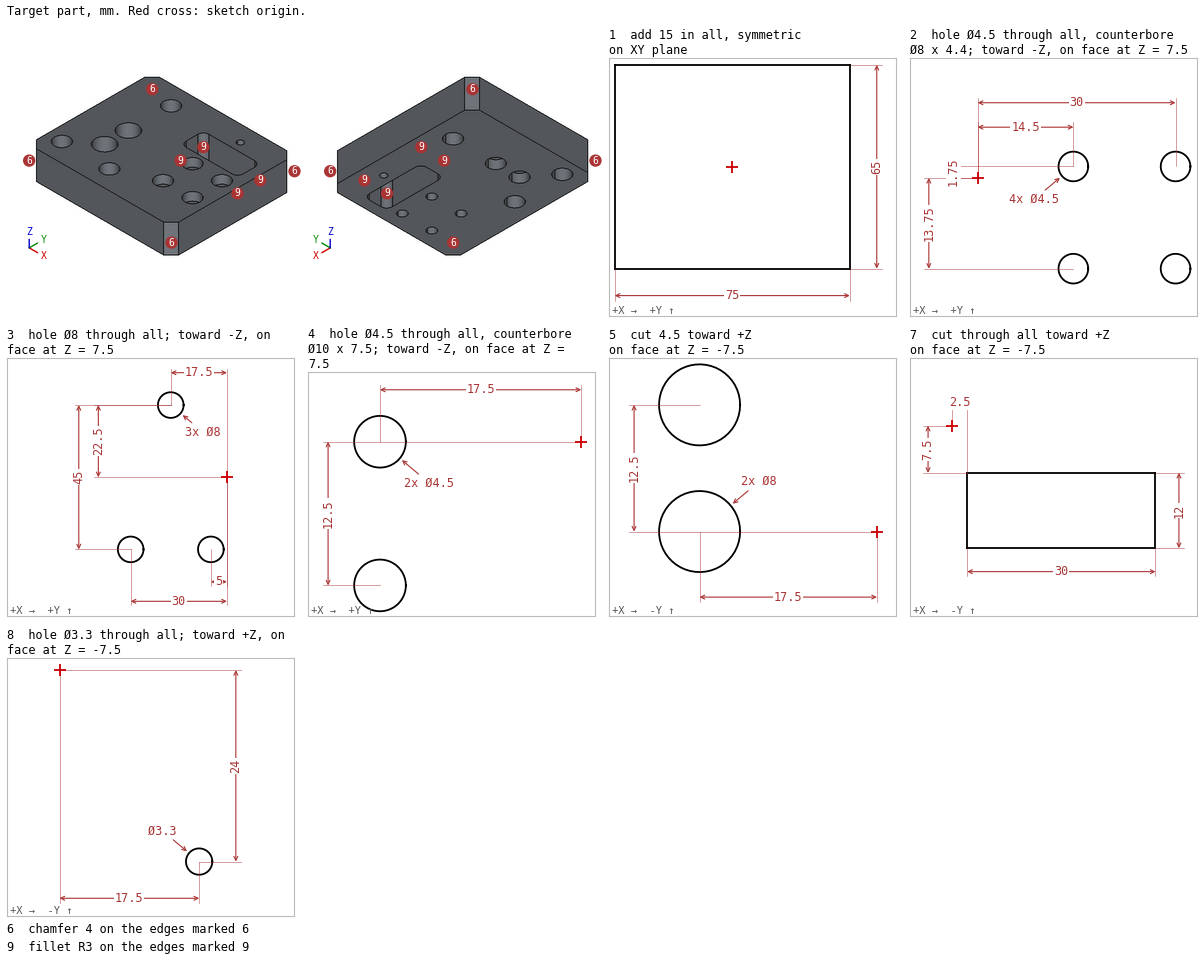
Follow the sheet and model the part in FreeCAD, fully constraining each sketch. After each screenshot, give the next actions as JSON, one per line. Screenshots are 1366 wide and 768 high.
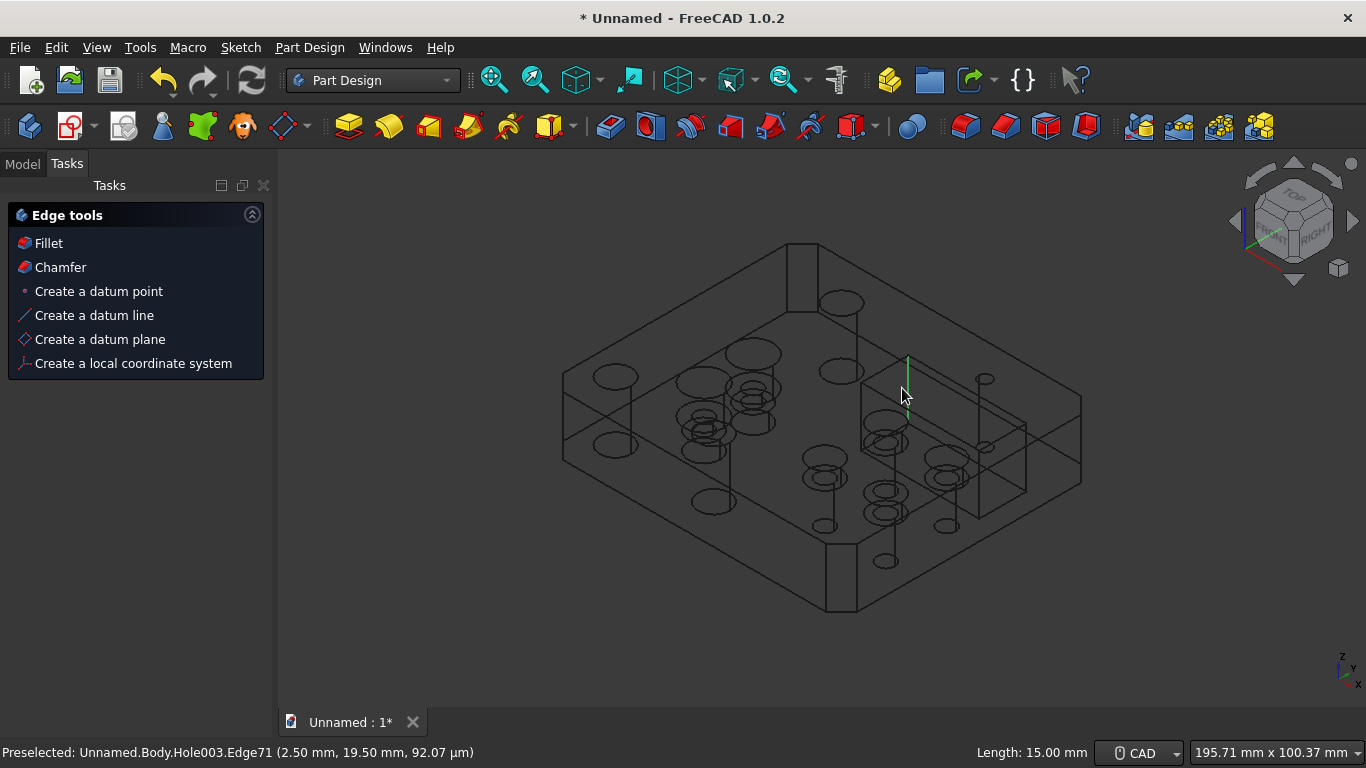
{"action": "left_click", "coordinate": [861, 409], "text": "ctrl"}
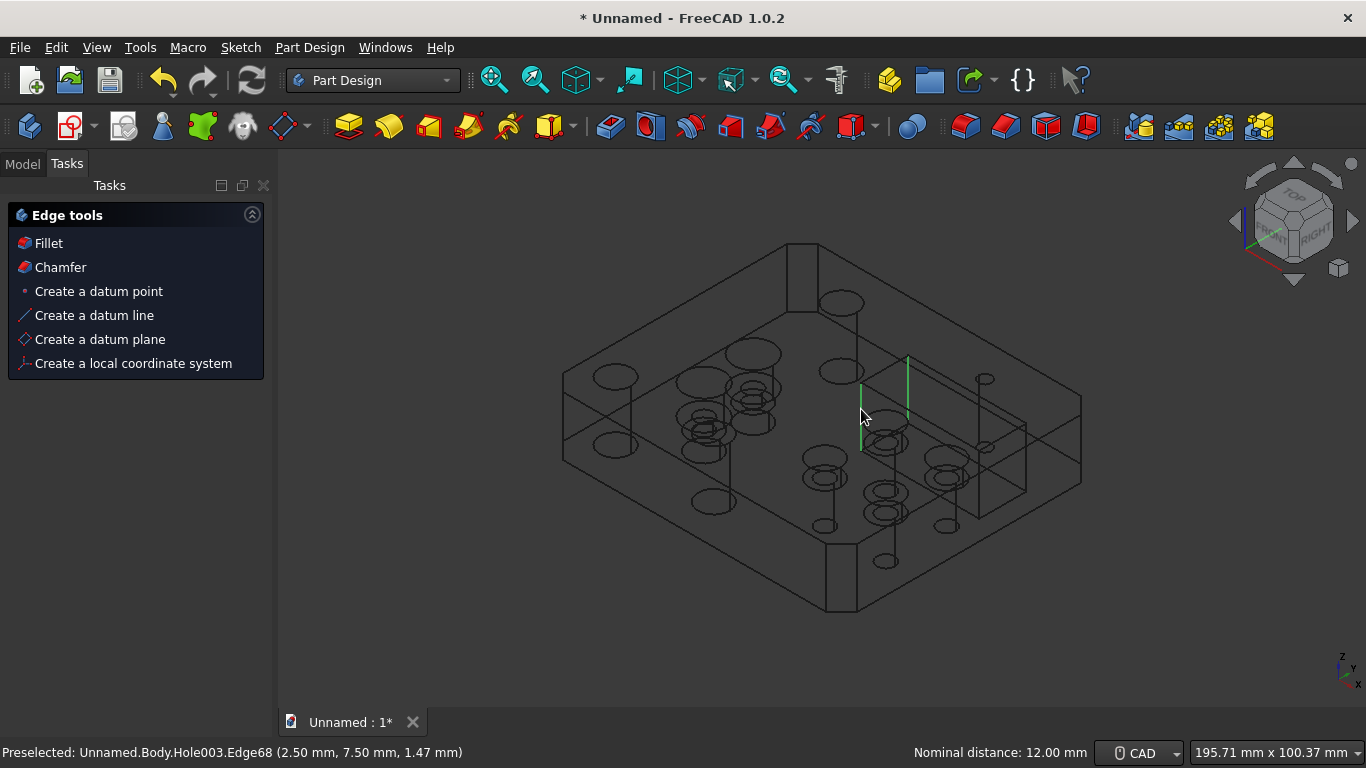
{"action": "left_click", "coordinate": [979, 484], "text": "ctrl"}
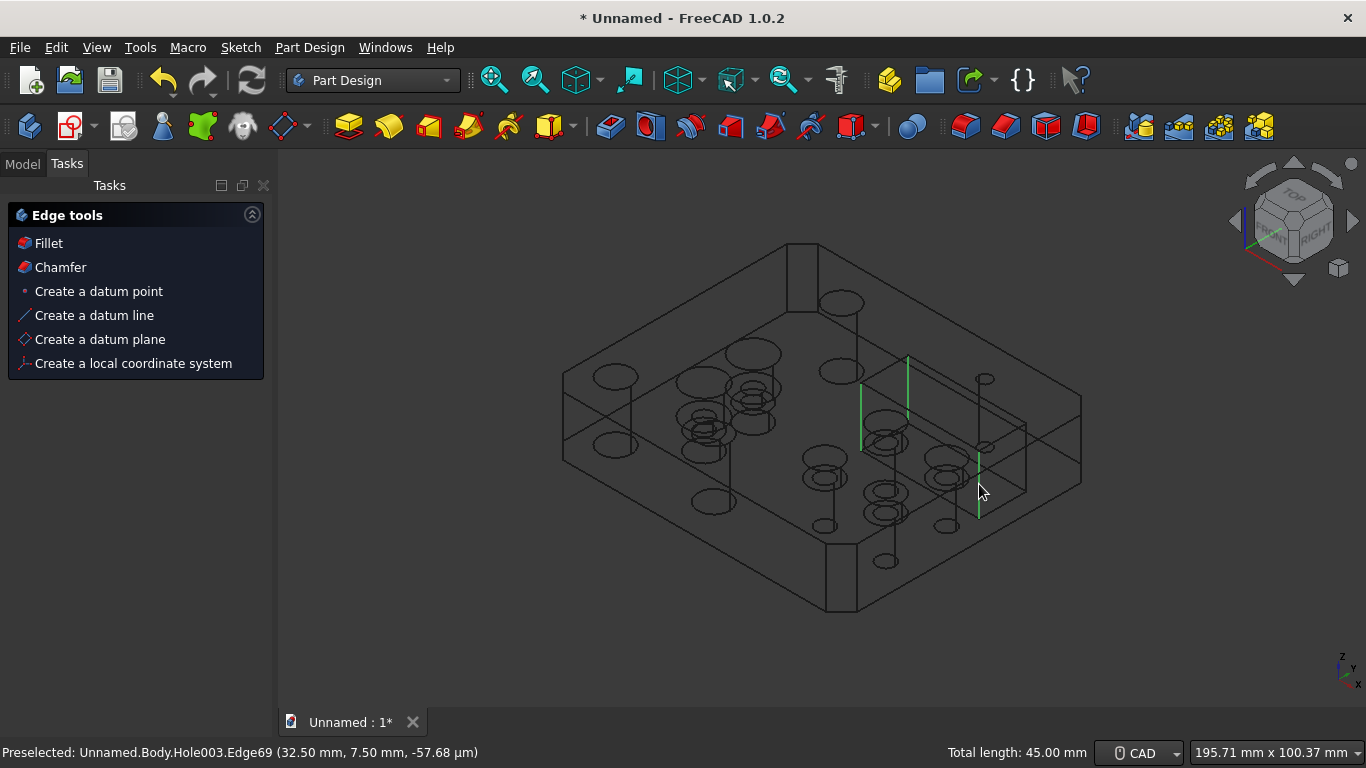
{"action": "left_click", "coordinate": [1026, 457], "text": "ctrl"}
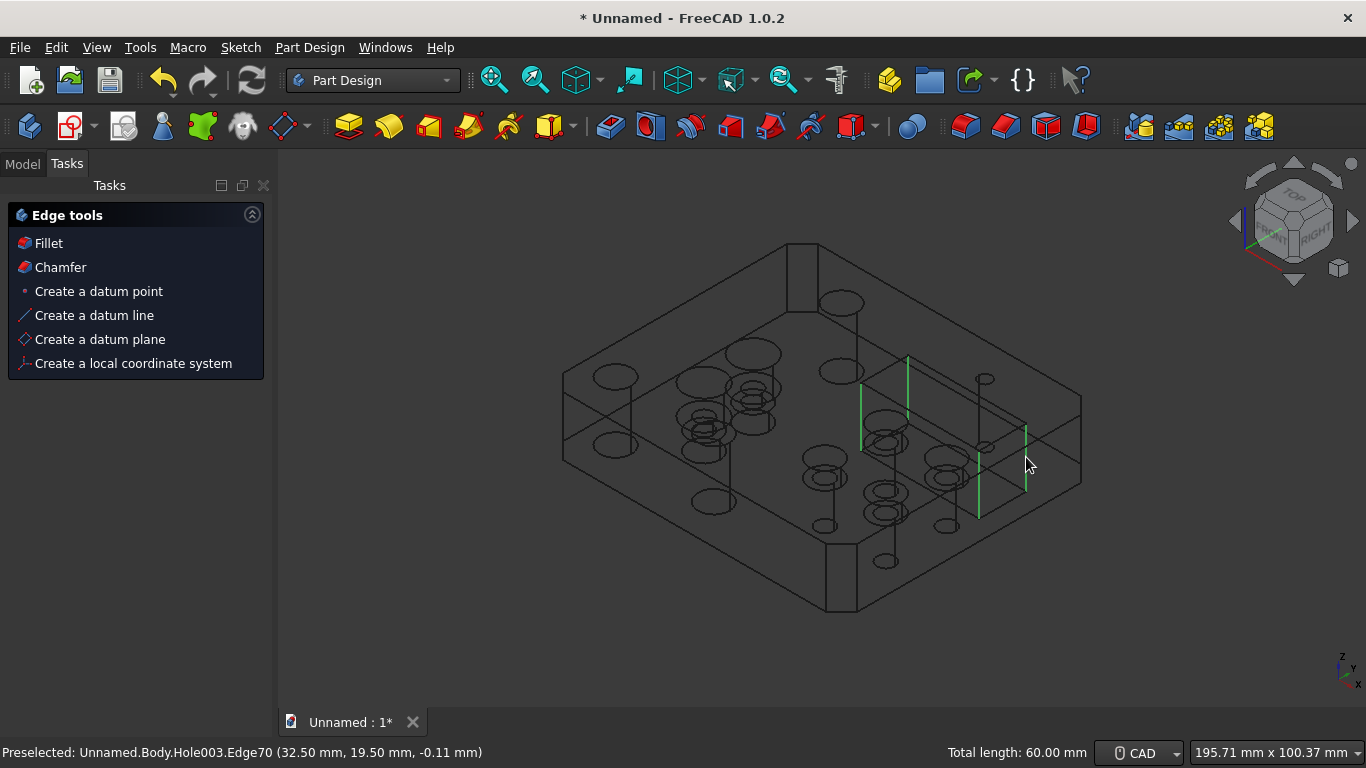
{"action": "key", "text": "v 1"}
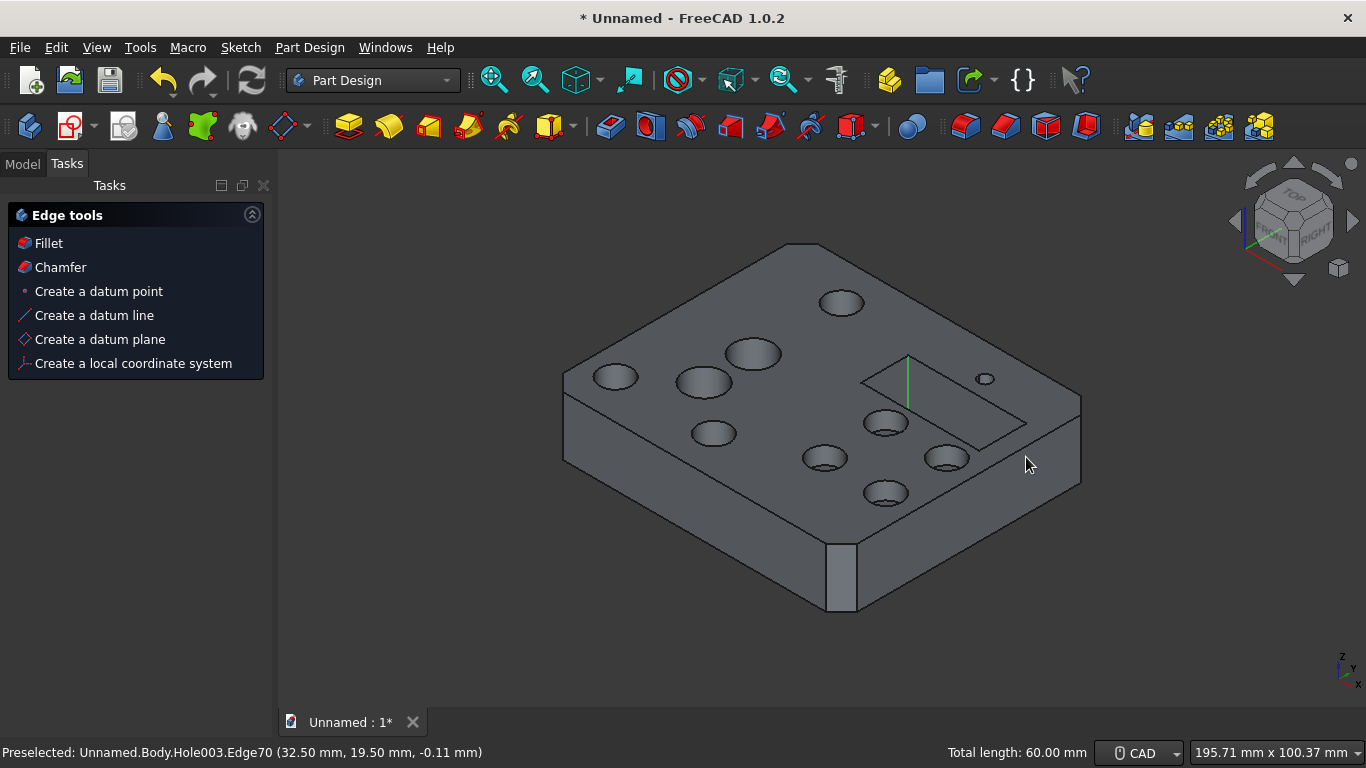
{"action": "left_click", "coordinate": [966, 126]}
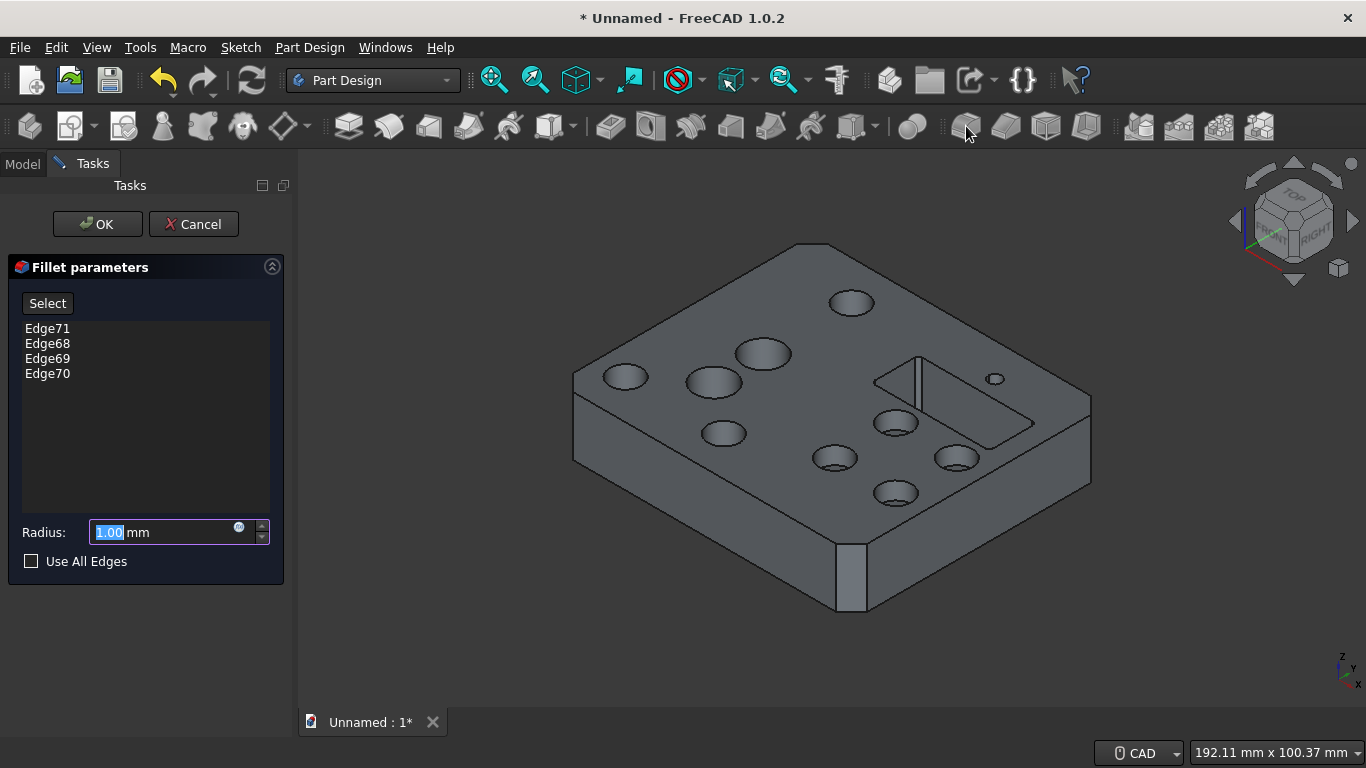
{"action": "type", "text": "3"}
{"action": "key", "text": "Tab"}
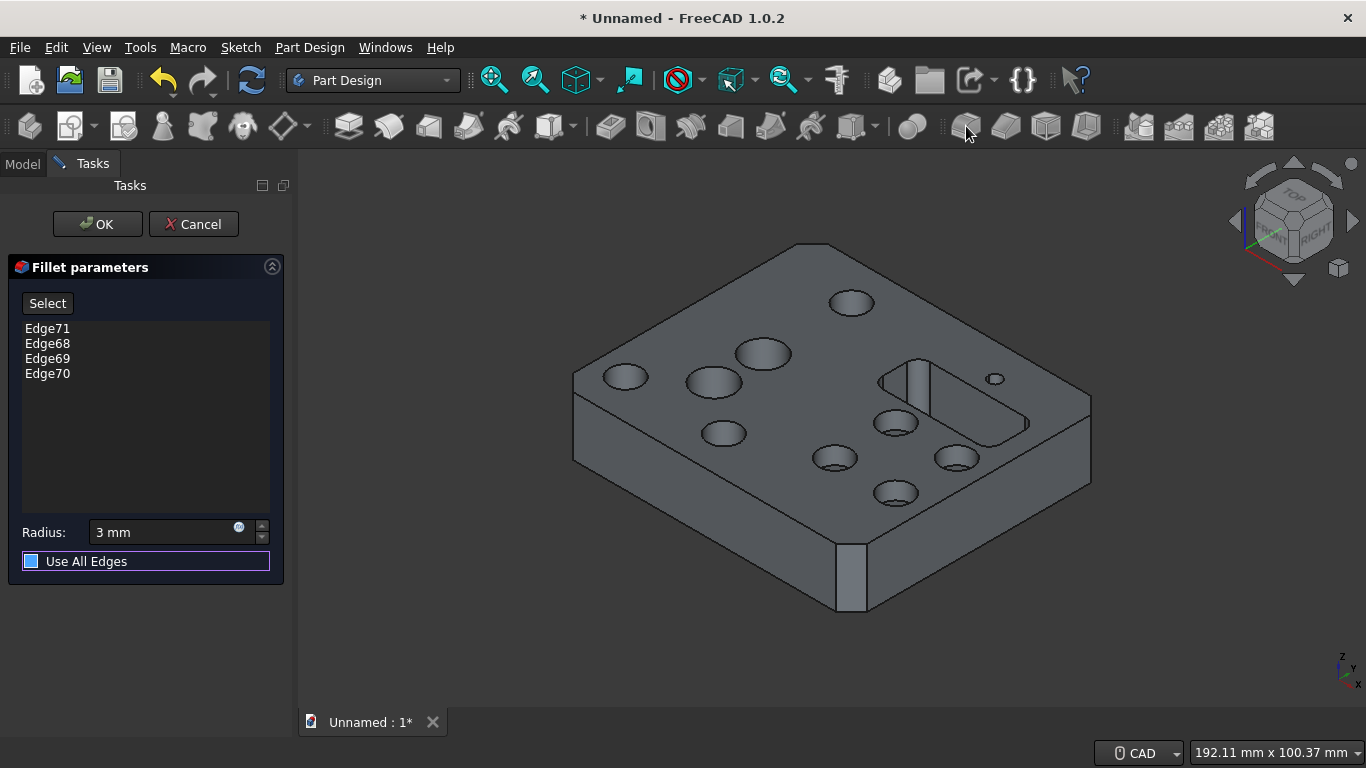
{"action": "left_click", "coordinate": [98, 224]}